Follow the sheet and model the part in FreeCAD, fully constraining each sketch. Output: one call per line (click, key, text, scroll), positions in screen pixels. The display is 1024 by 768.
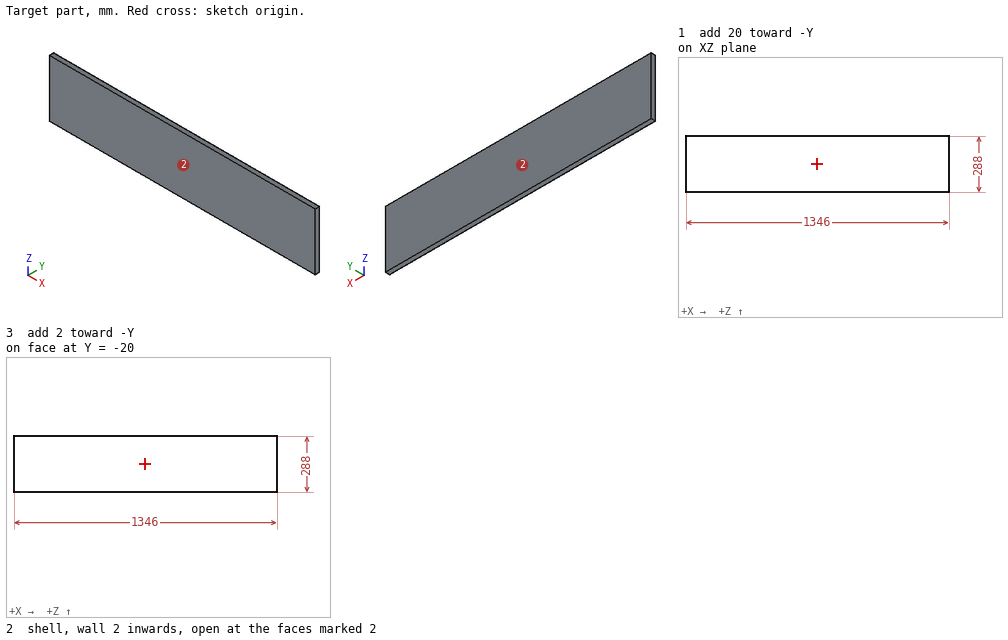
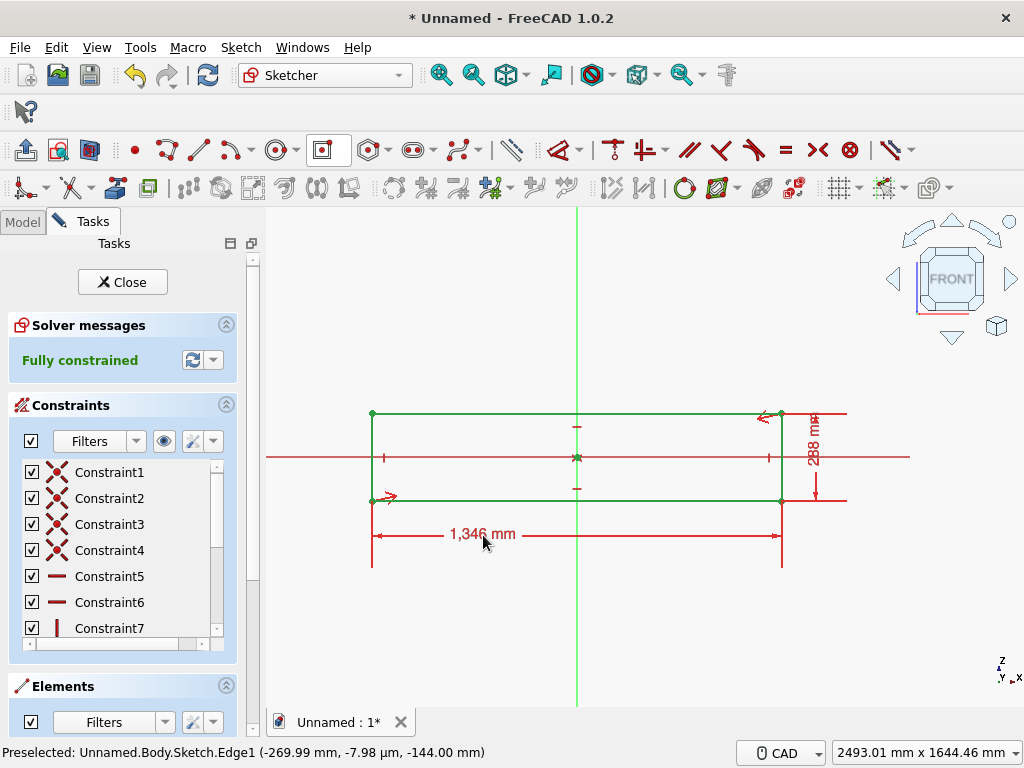
click(123, 282)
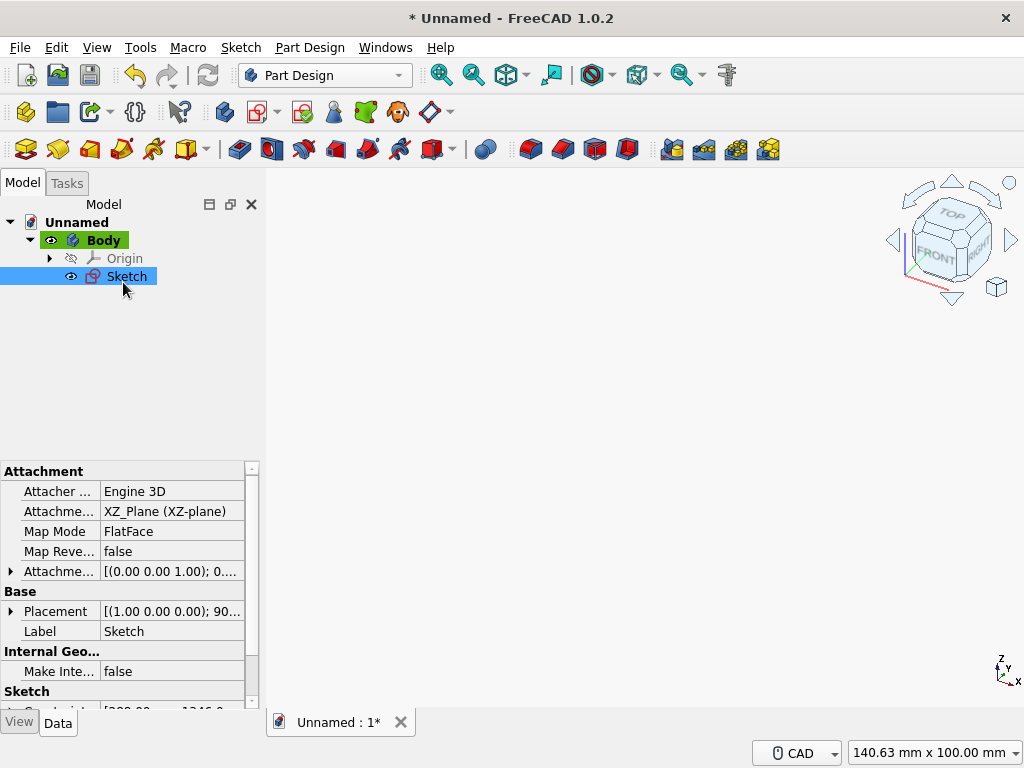
click(26, 150)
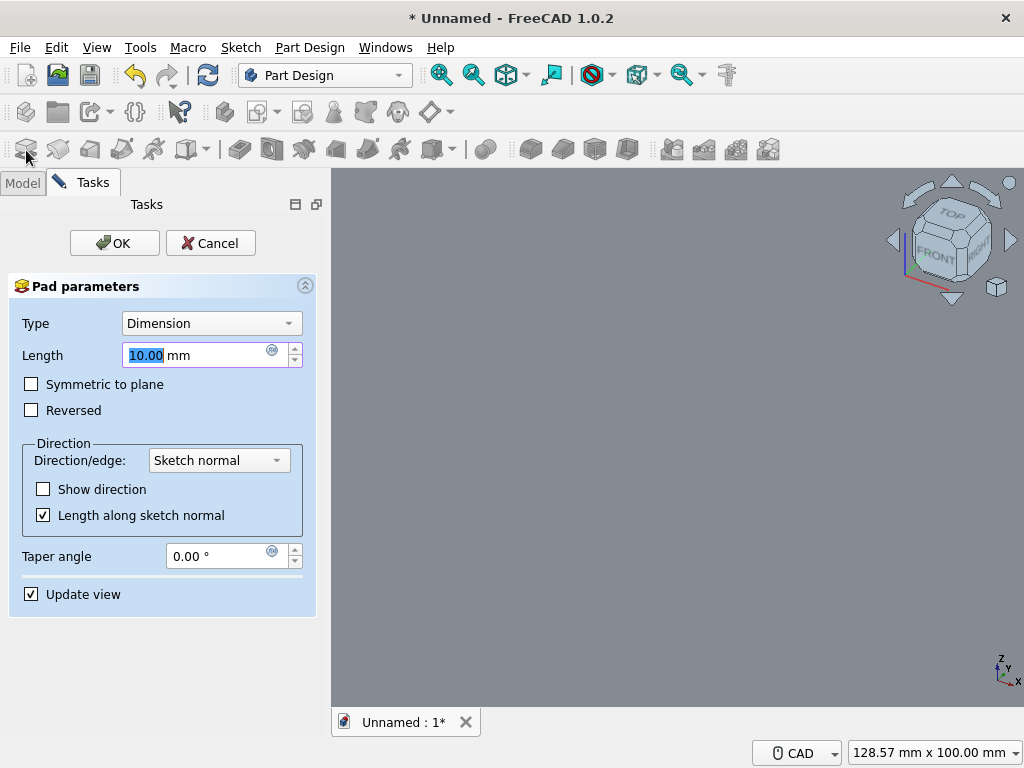
text(20)
key(Tab)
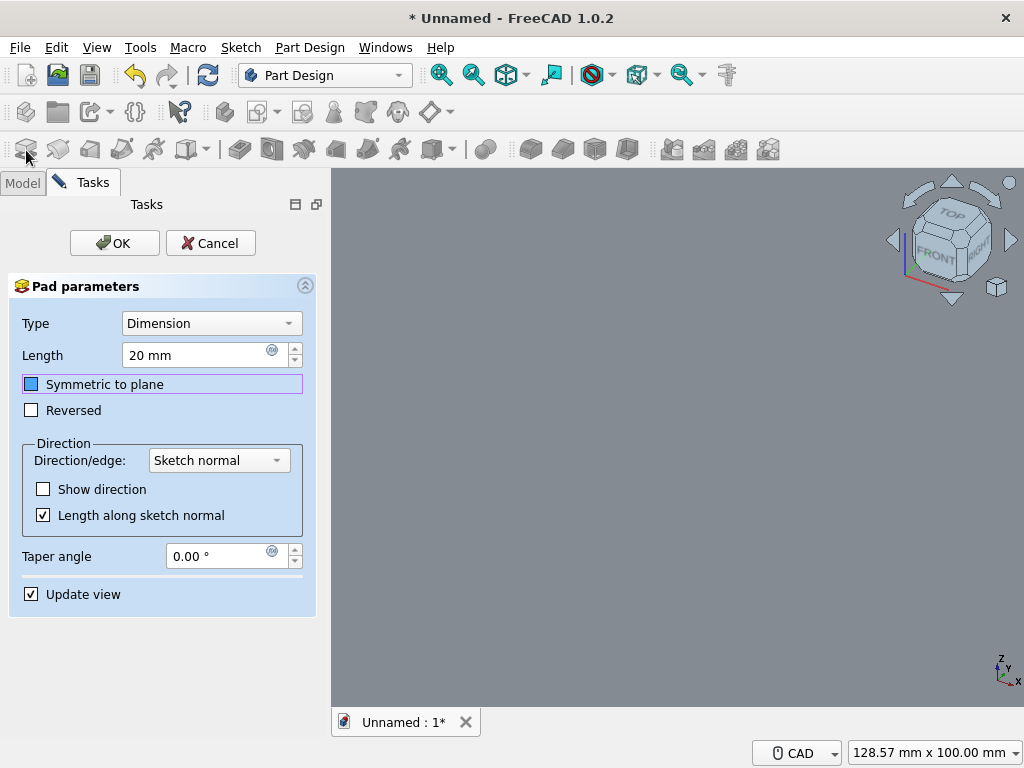
click(115, 243)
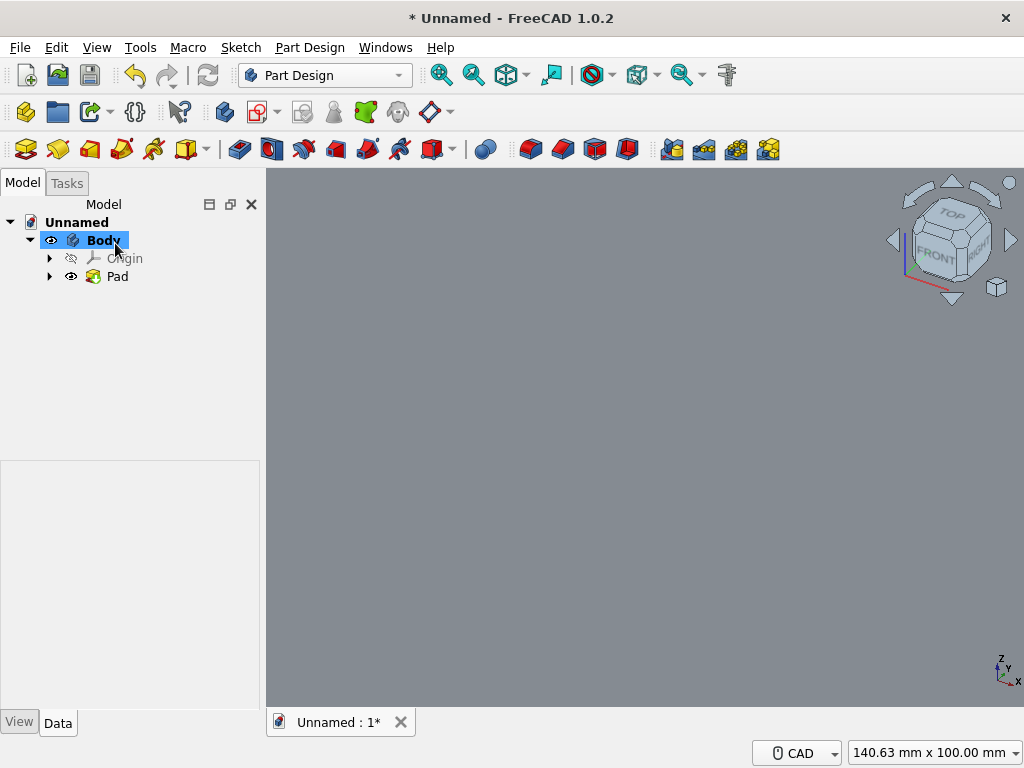
click(442, 76)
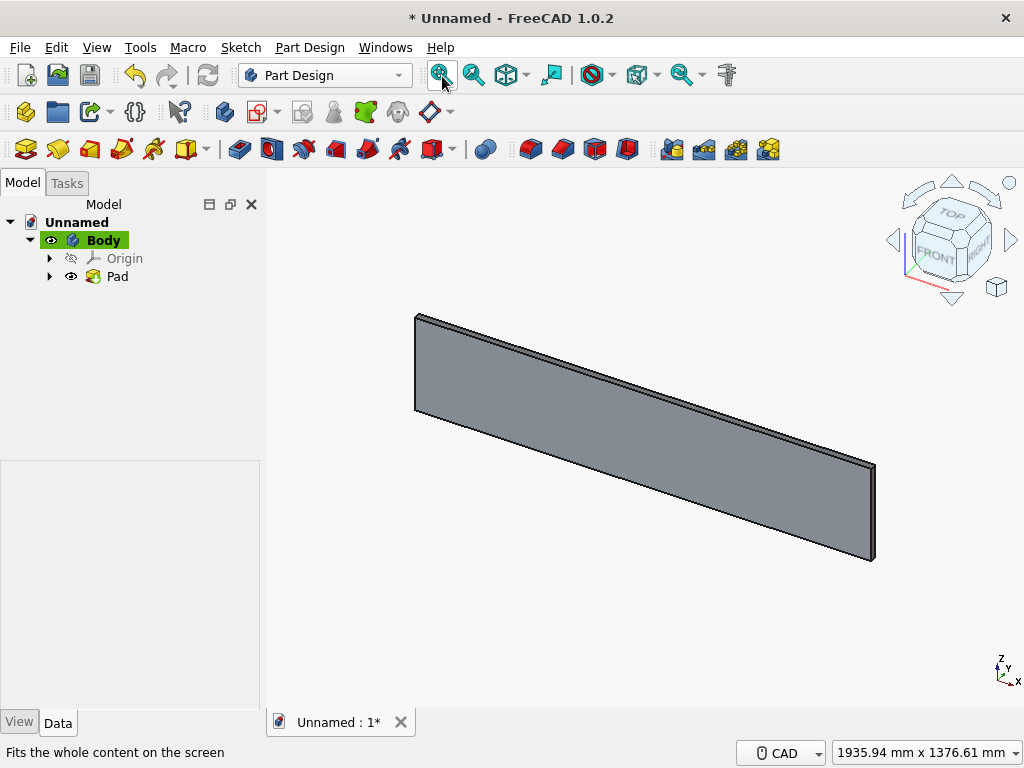
click(773, 482)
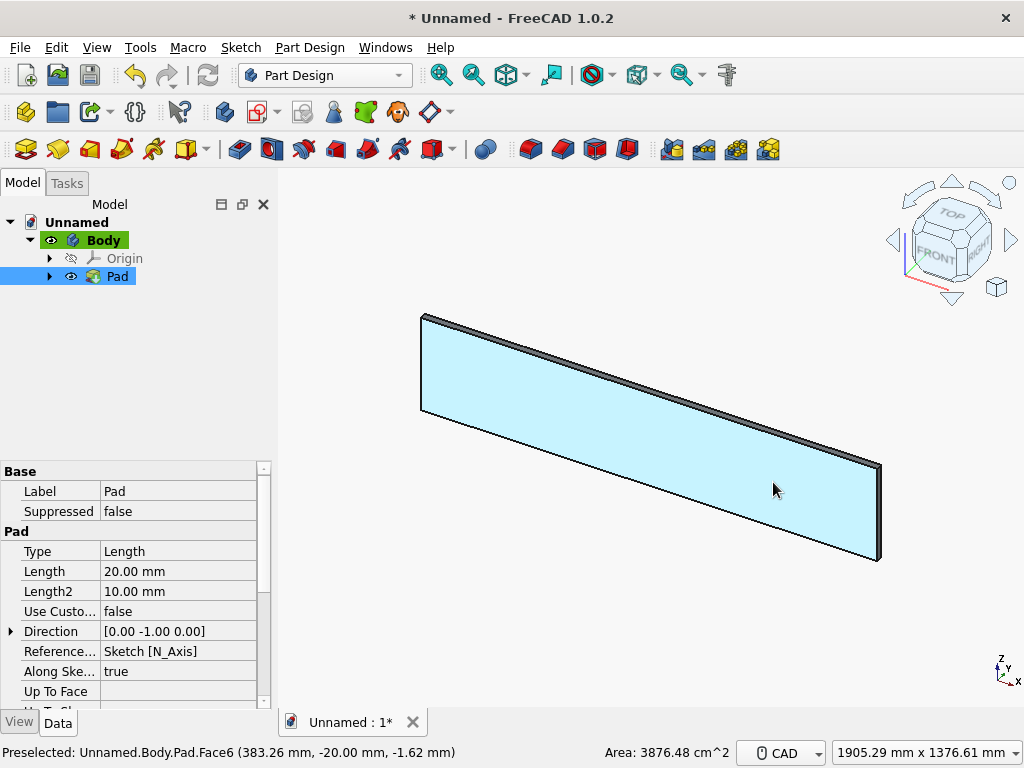
click(628, 150)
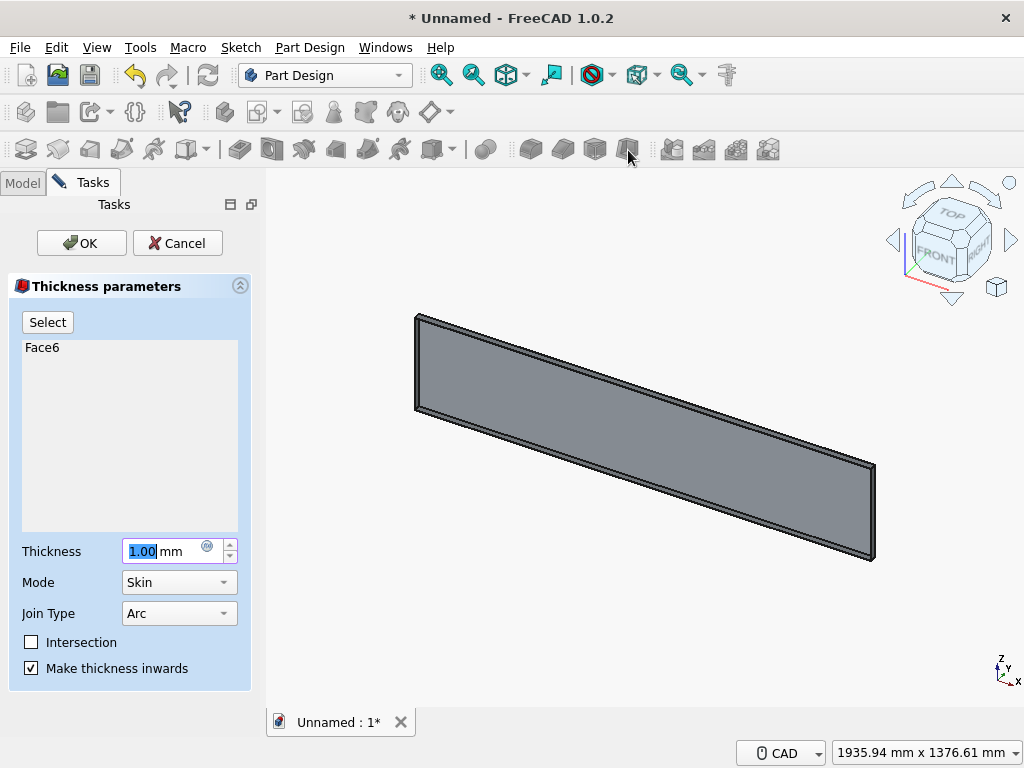
text(2)
key(Tab)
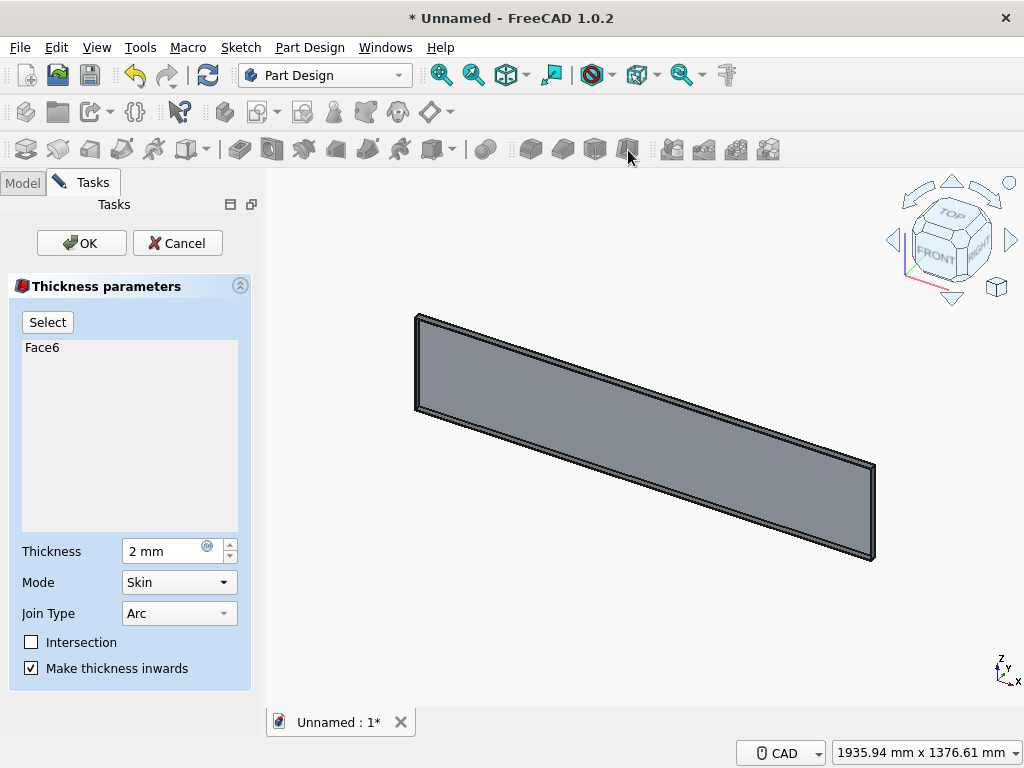
click(180, 614)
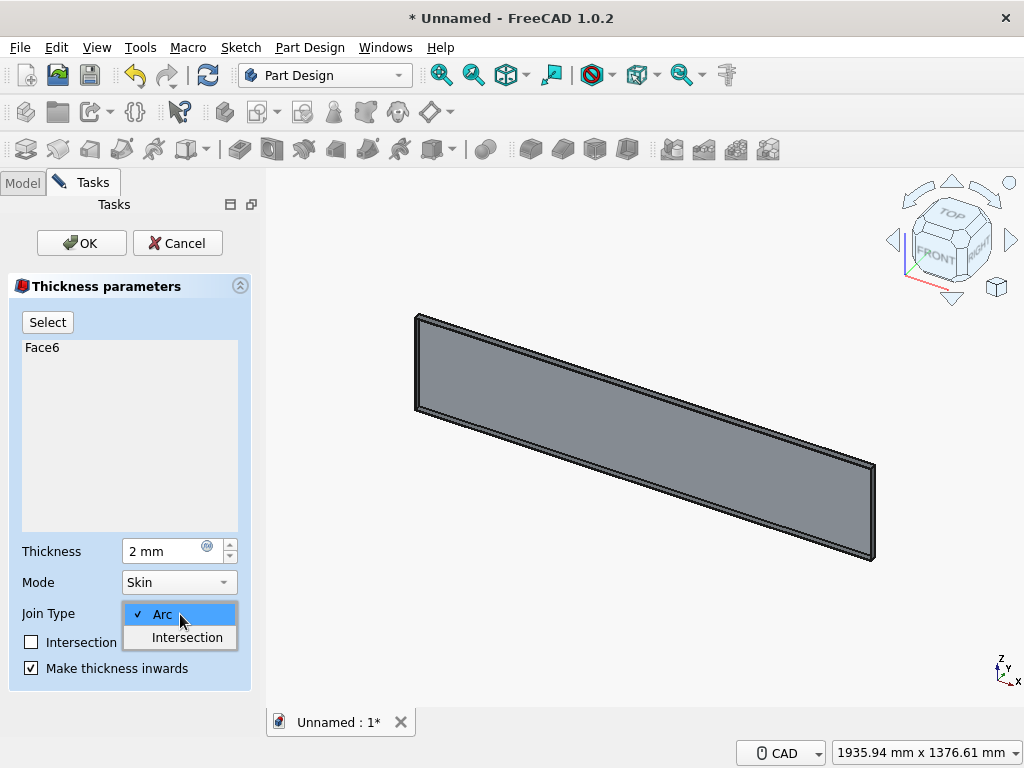
click(179, 638)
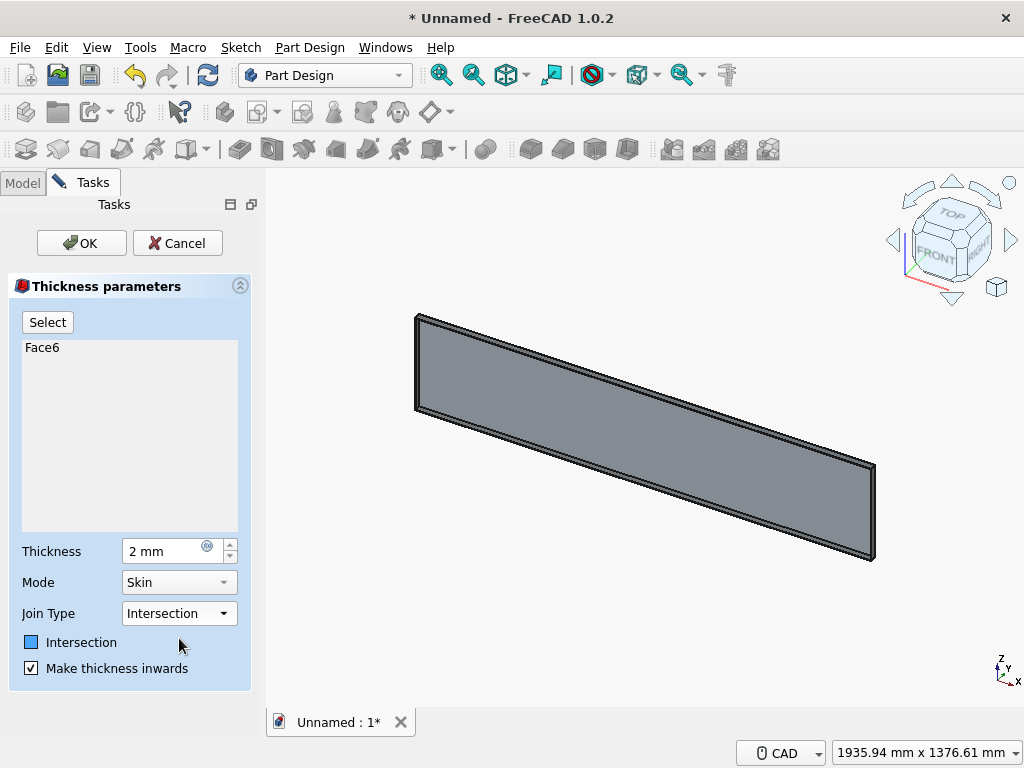
click(82, 243)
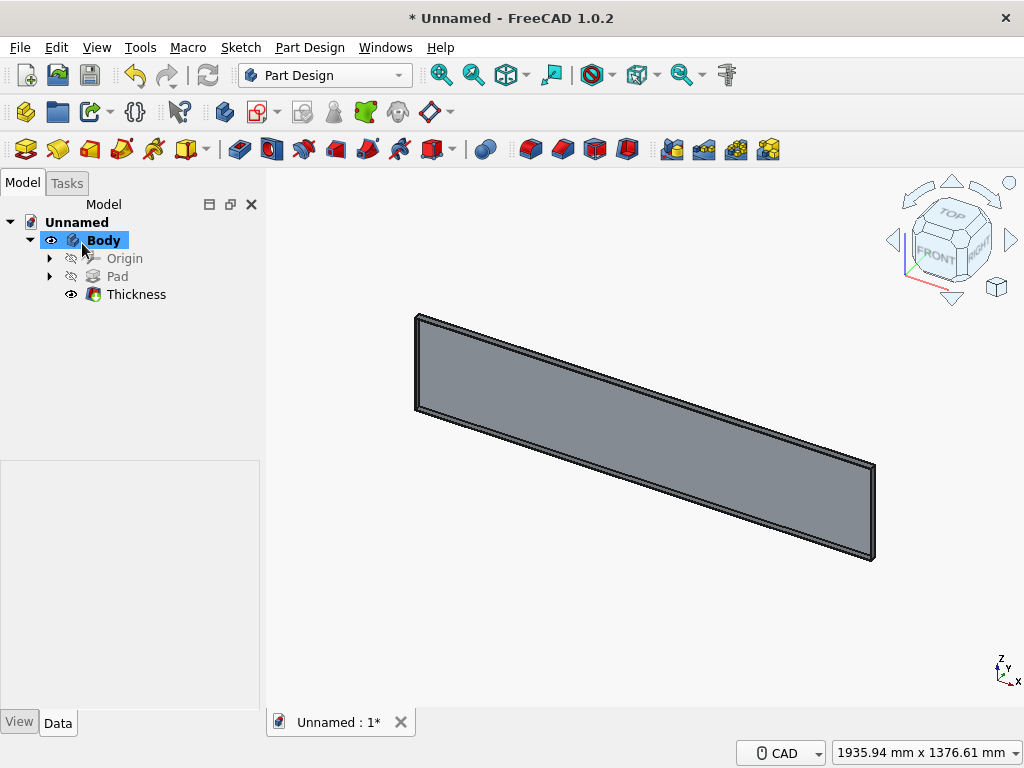
key(0)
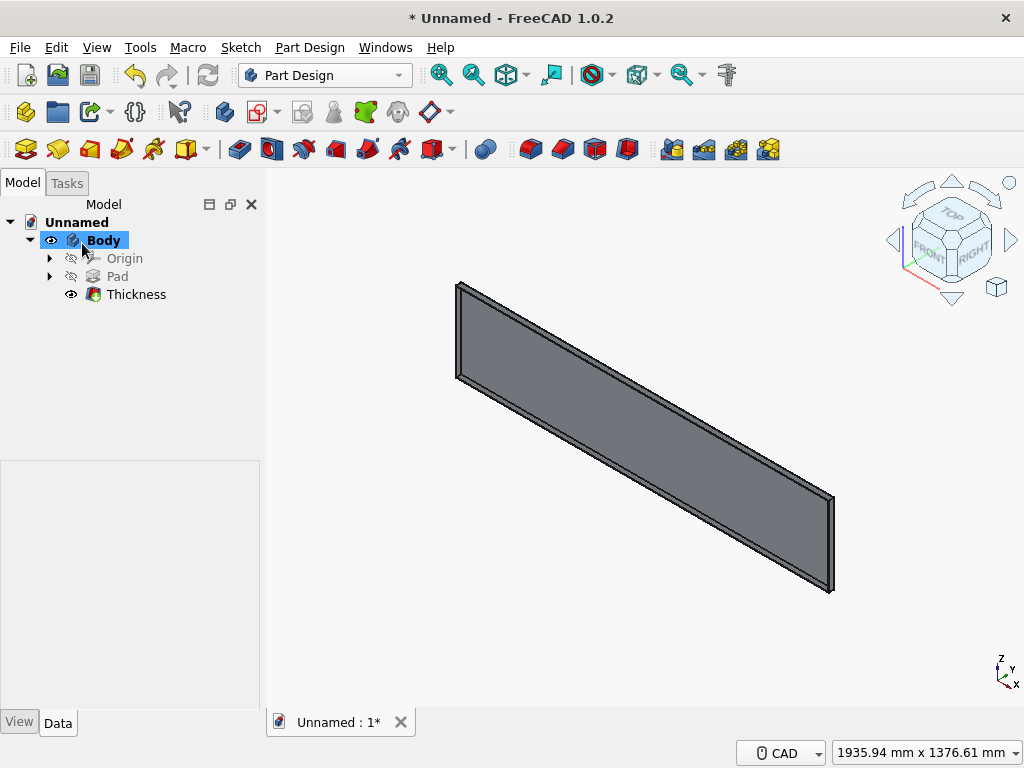
scroll(828, 530, up, 15)